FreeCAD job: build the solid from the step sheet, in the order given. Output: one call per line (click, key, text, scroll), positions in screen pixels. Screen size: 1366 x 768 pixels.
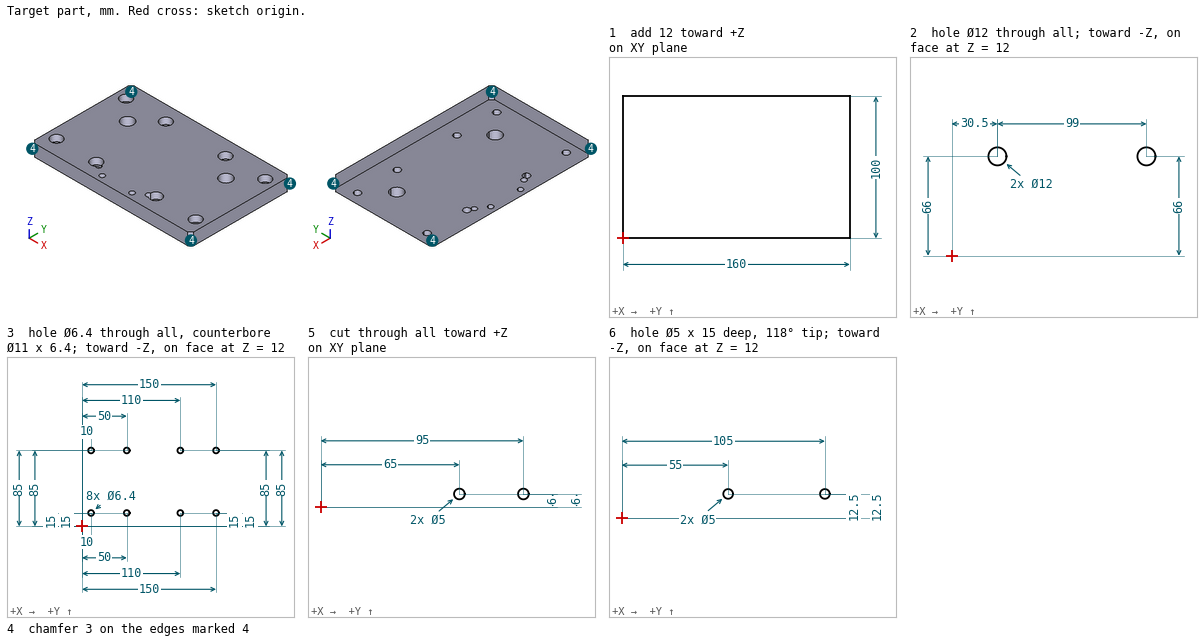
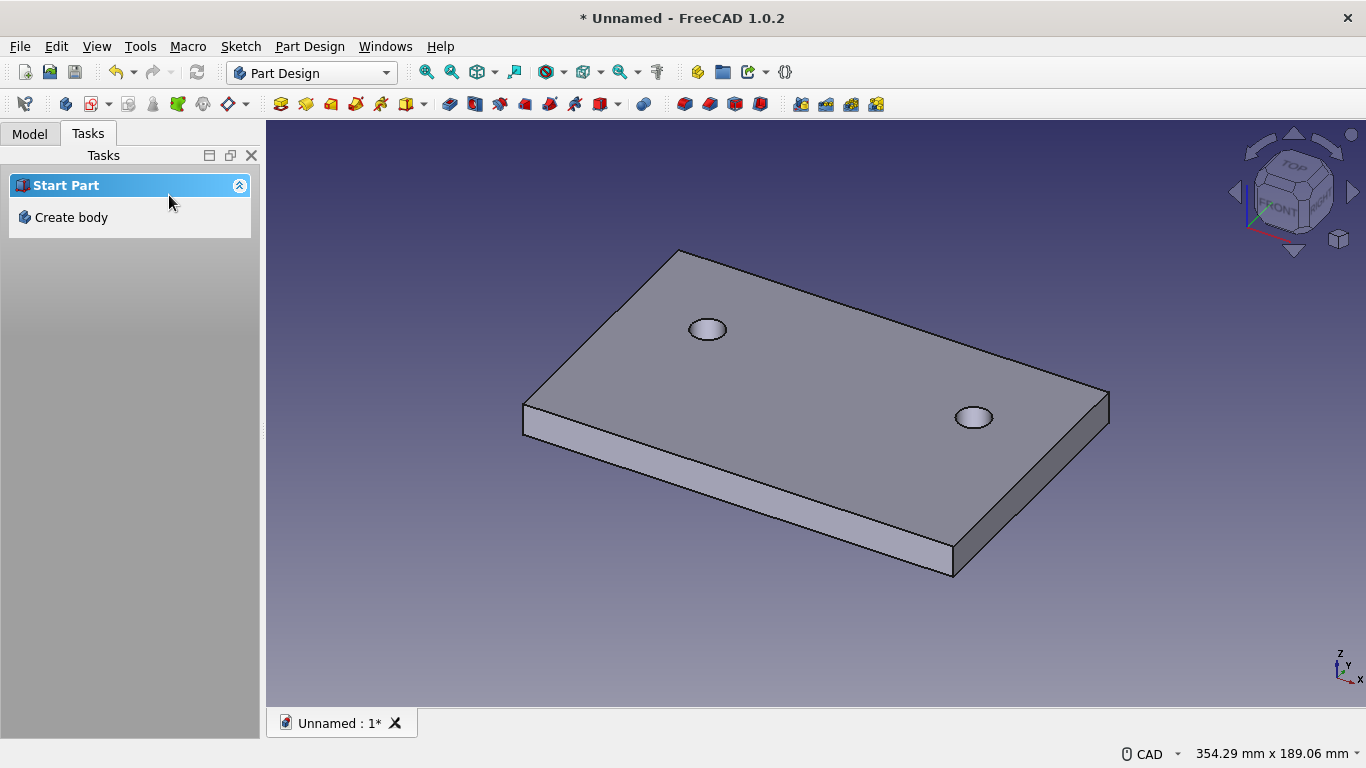
click(816, 397)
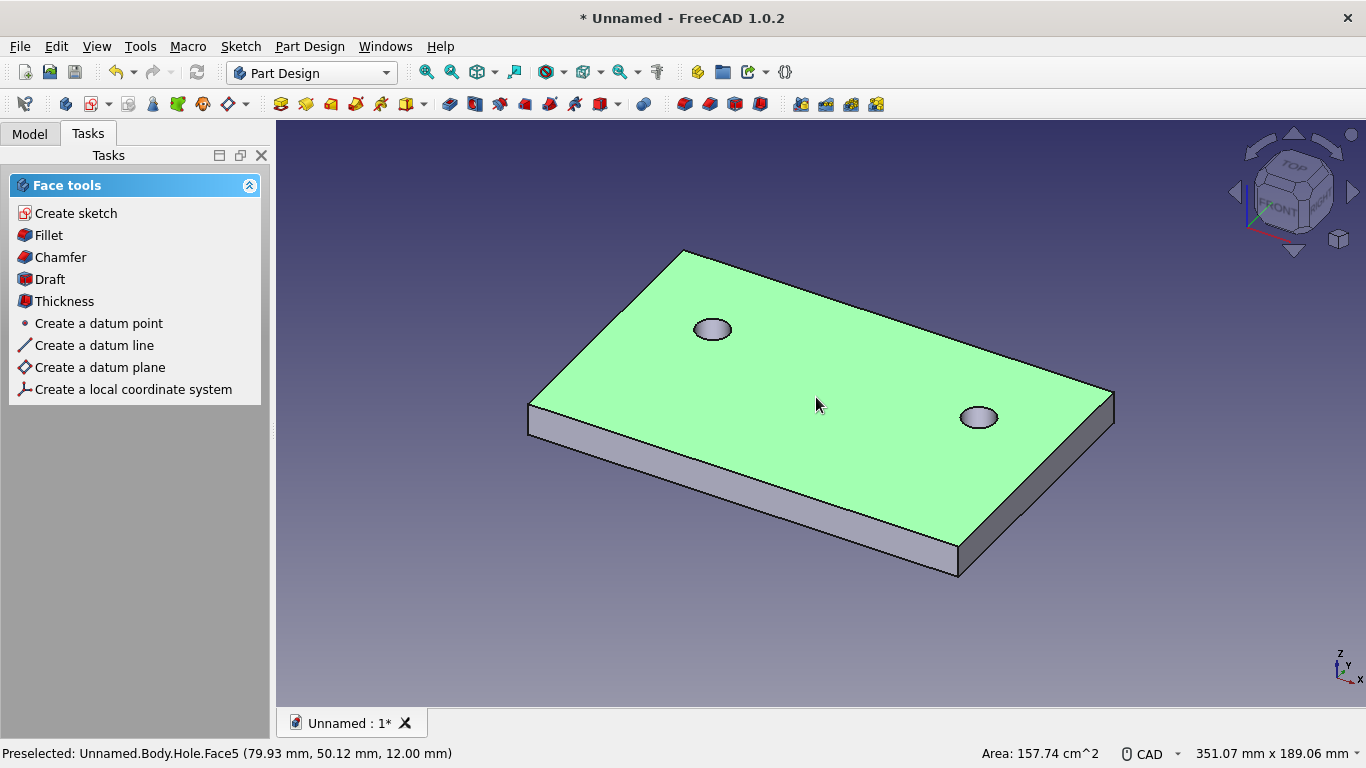
click(90, 104)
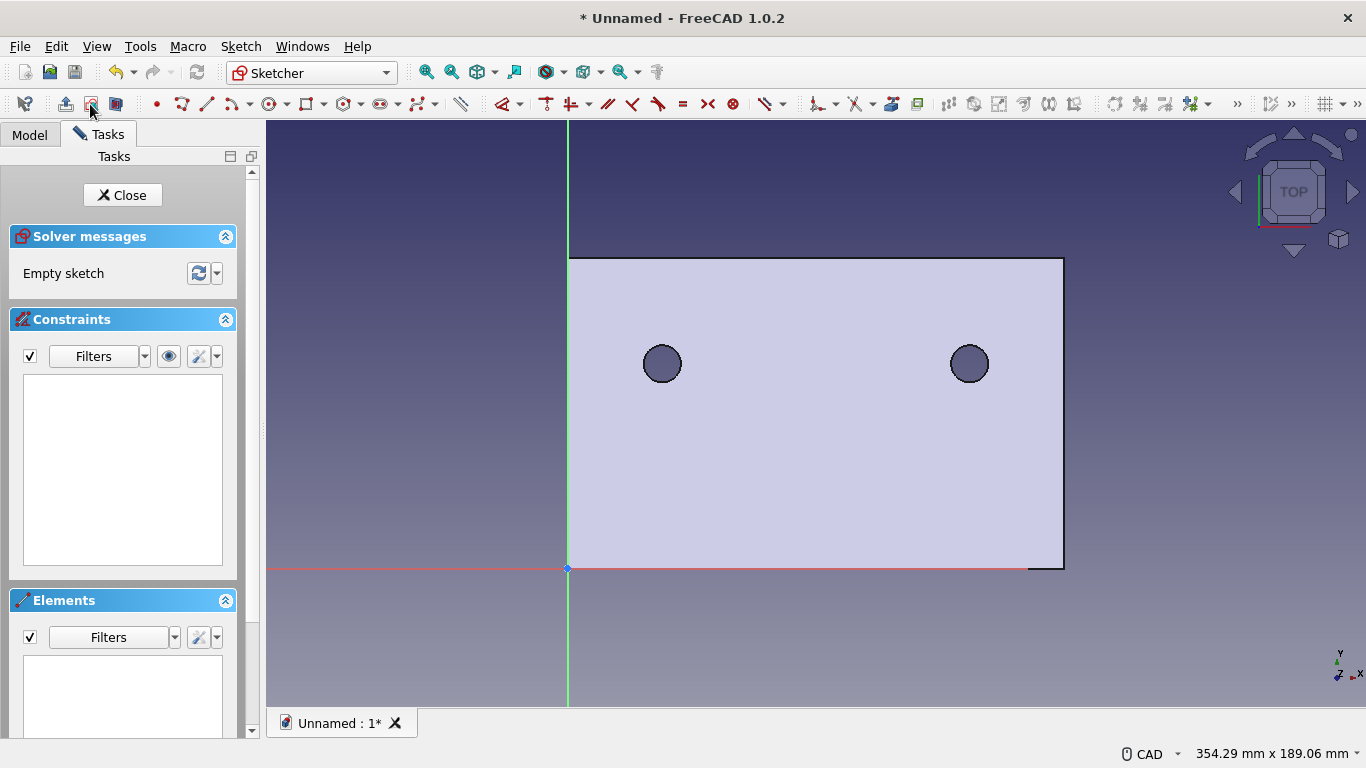
key(g)
key(c)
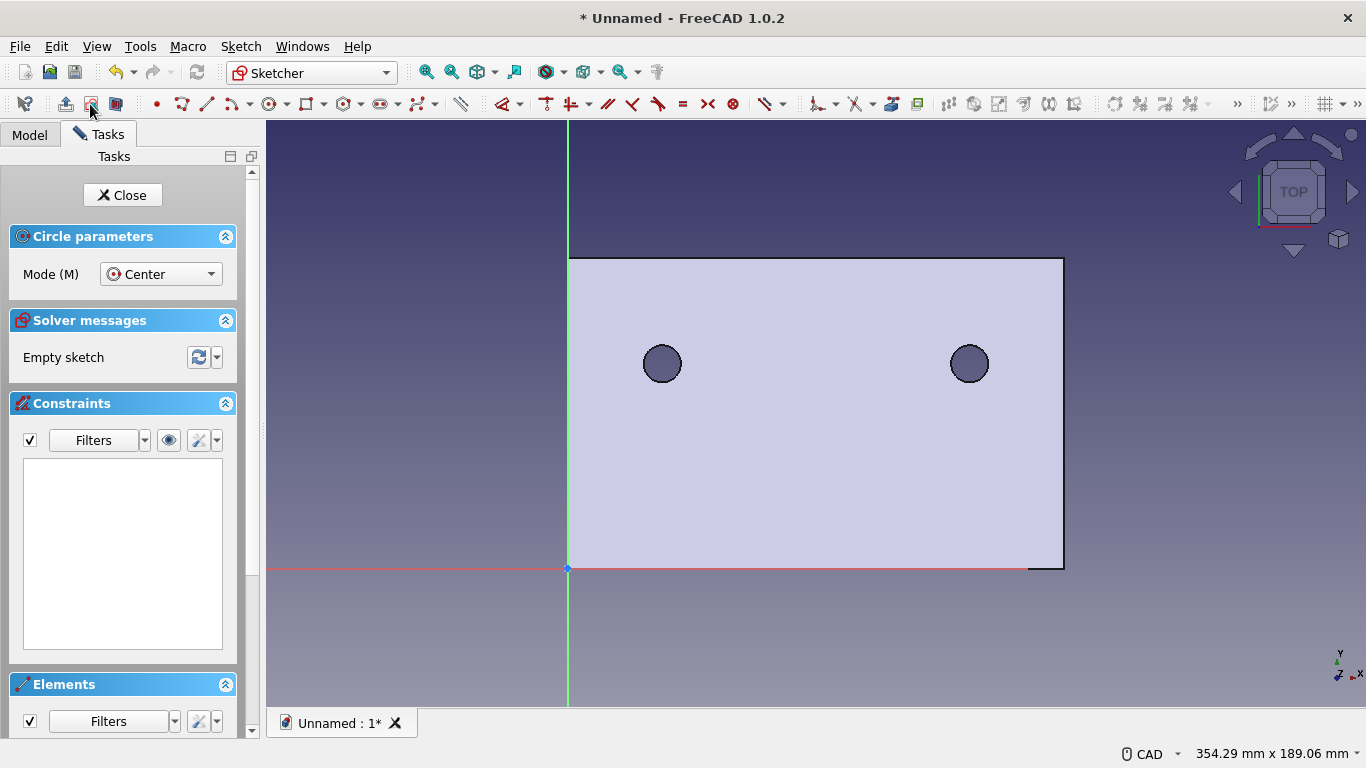
scroll(599, 522, up, 5)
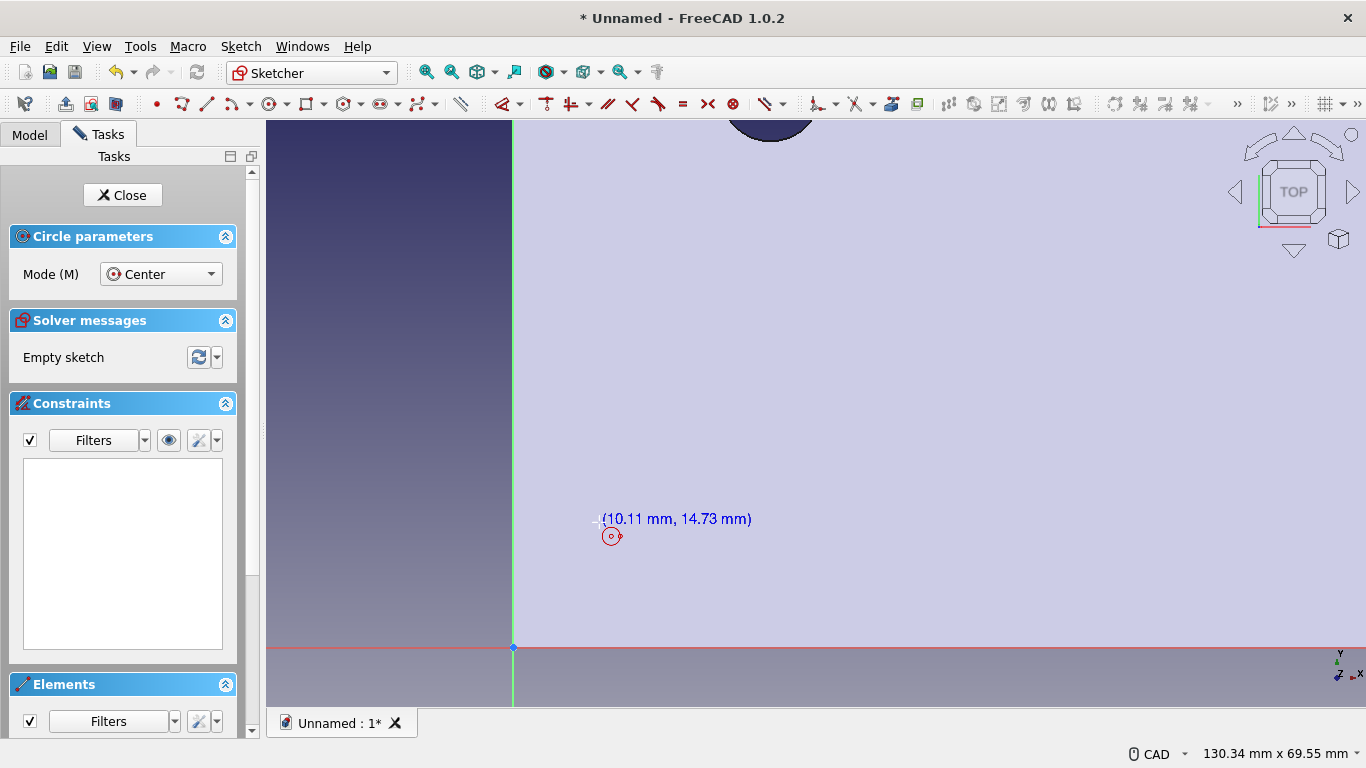
click(598, 521)
click(617, 502)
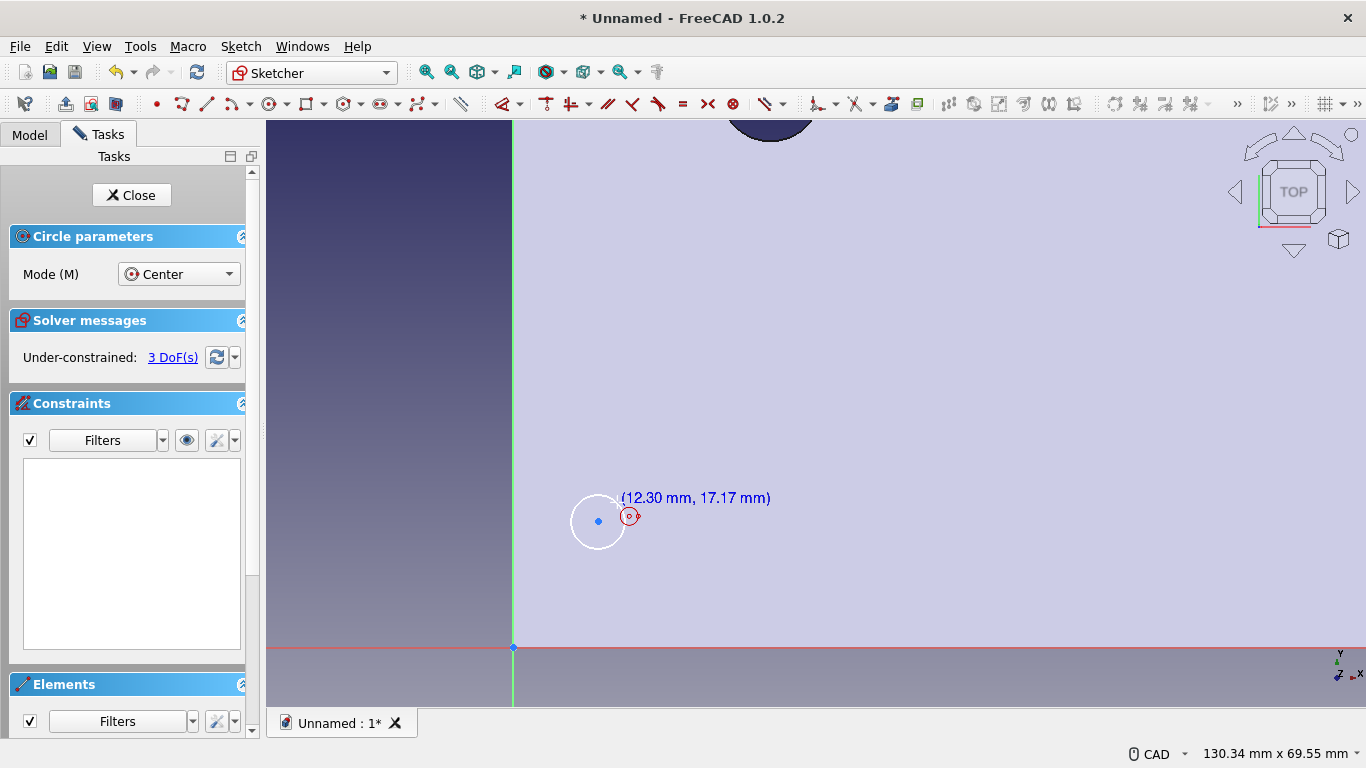
click(935, 521)
click(954, 502)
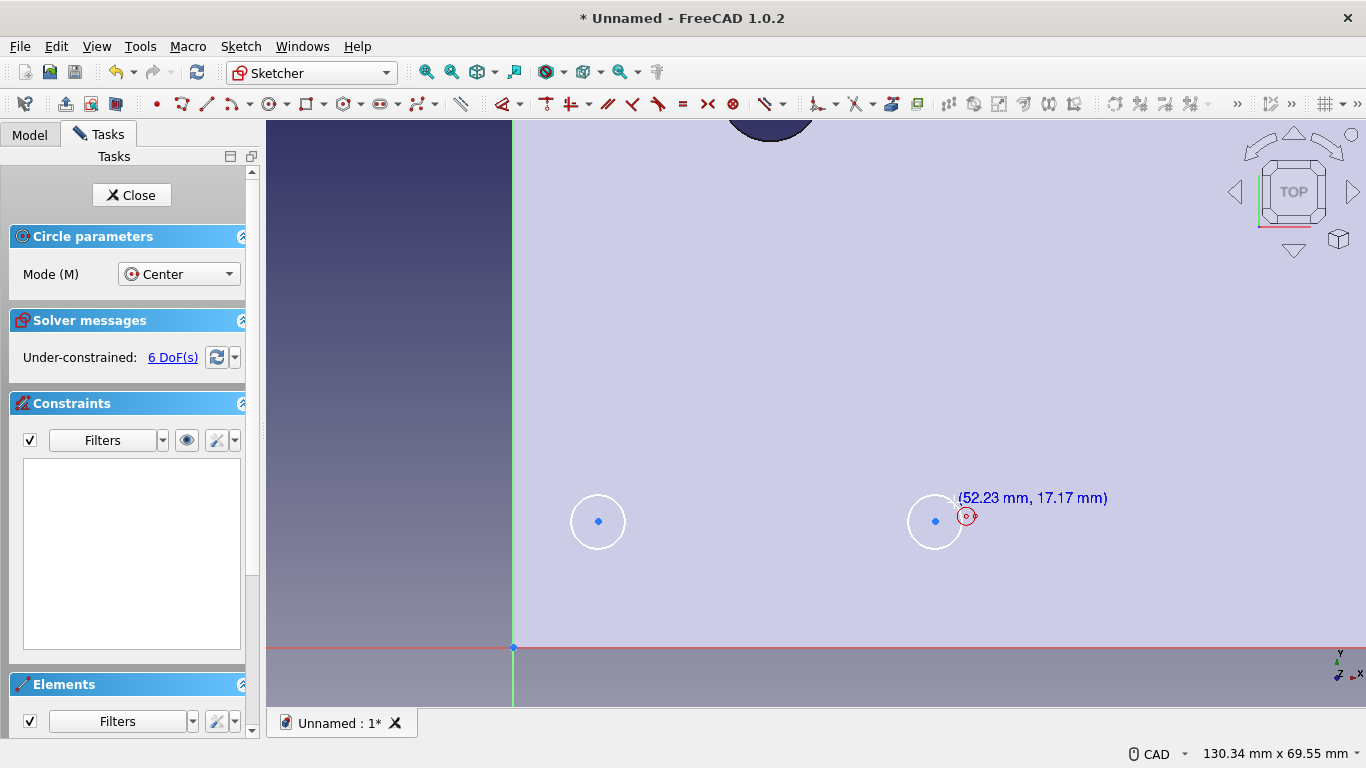
scroll(411, 526, down, 4)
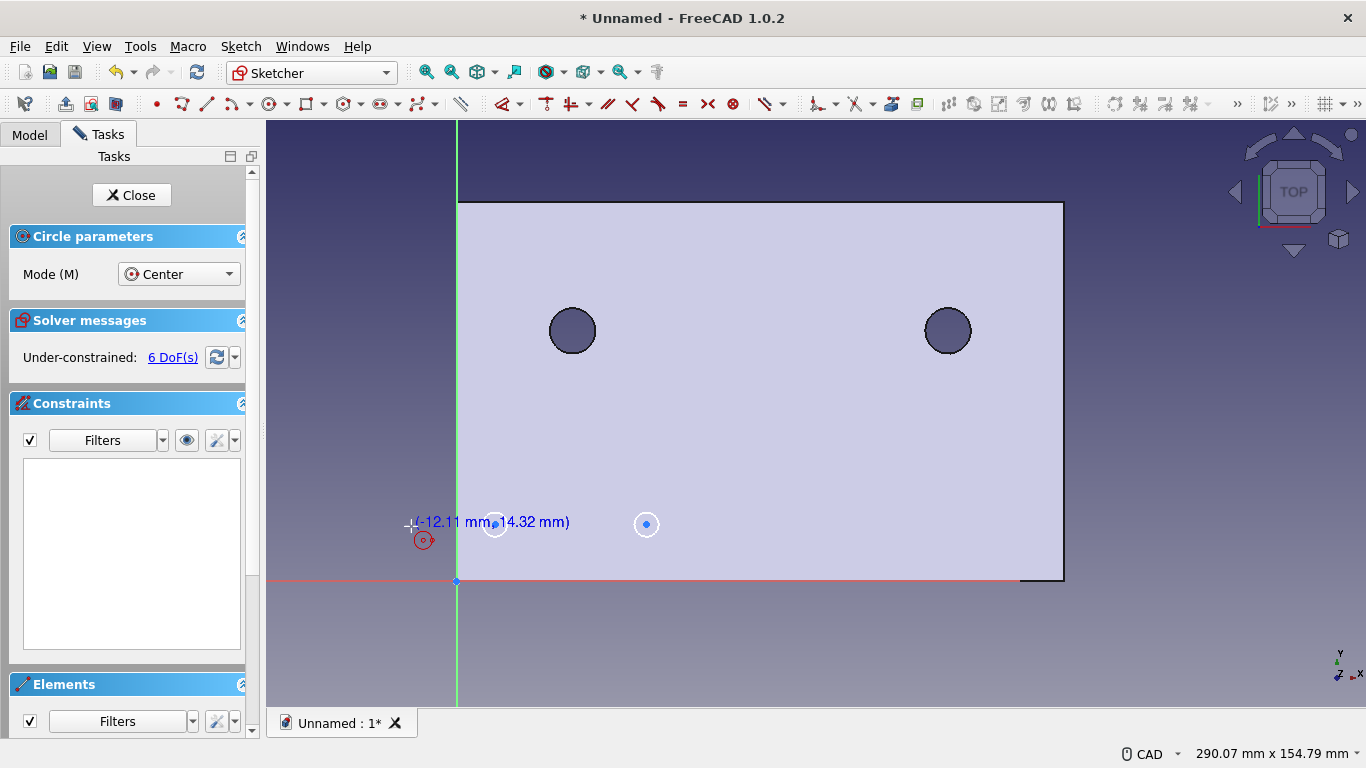
scroll(647, 259, up, 4)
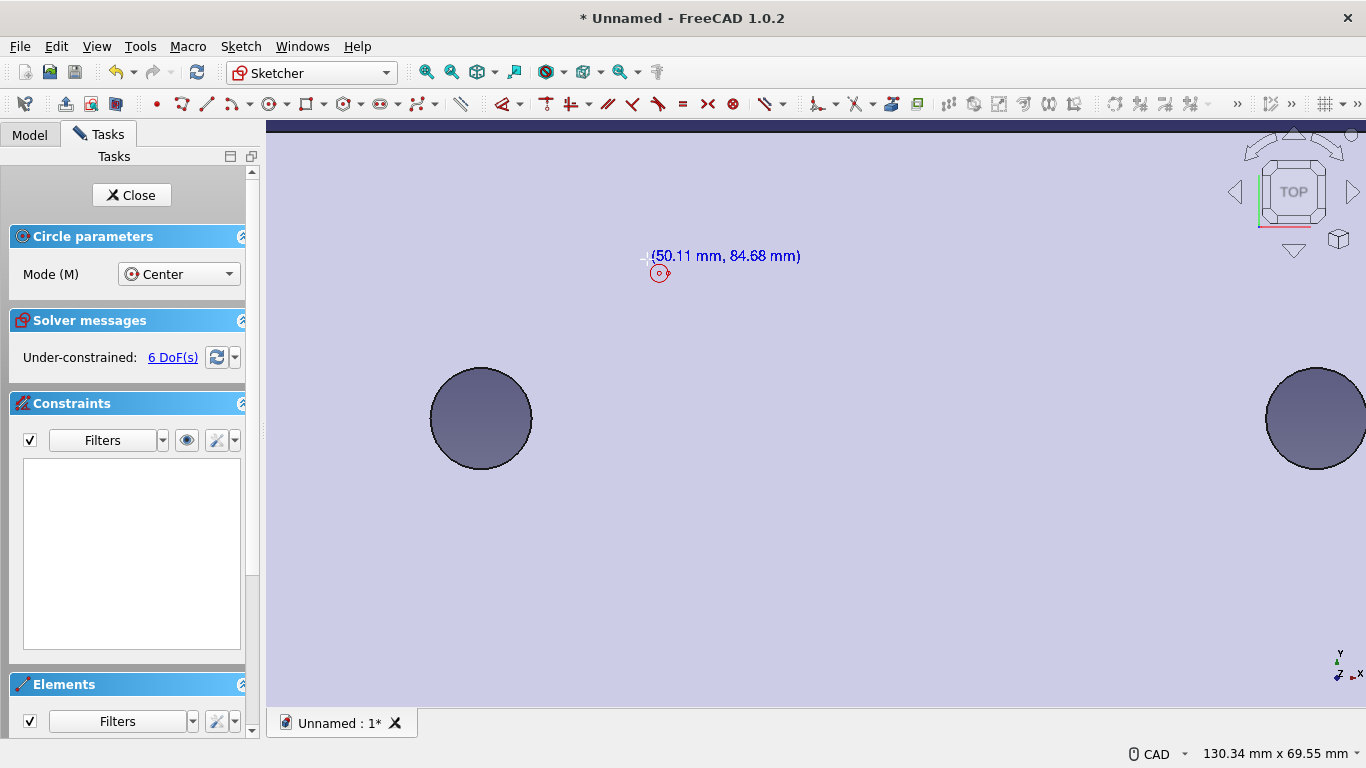
click(646, 258)
click(665, 239)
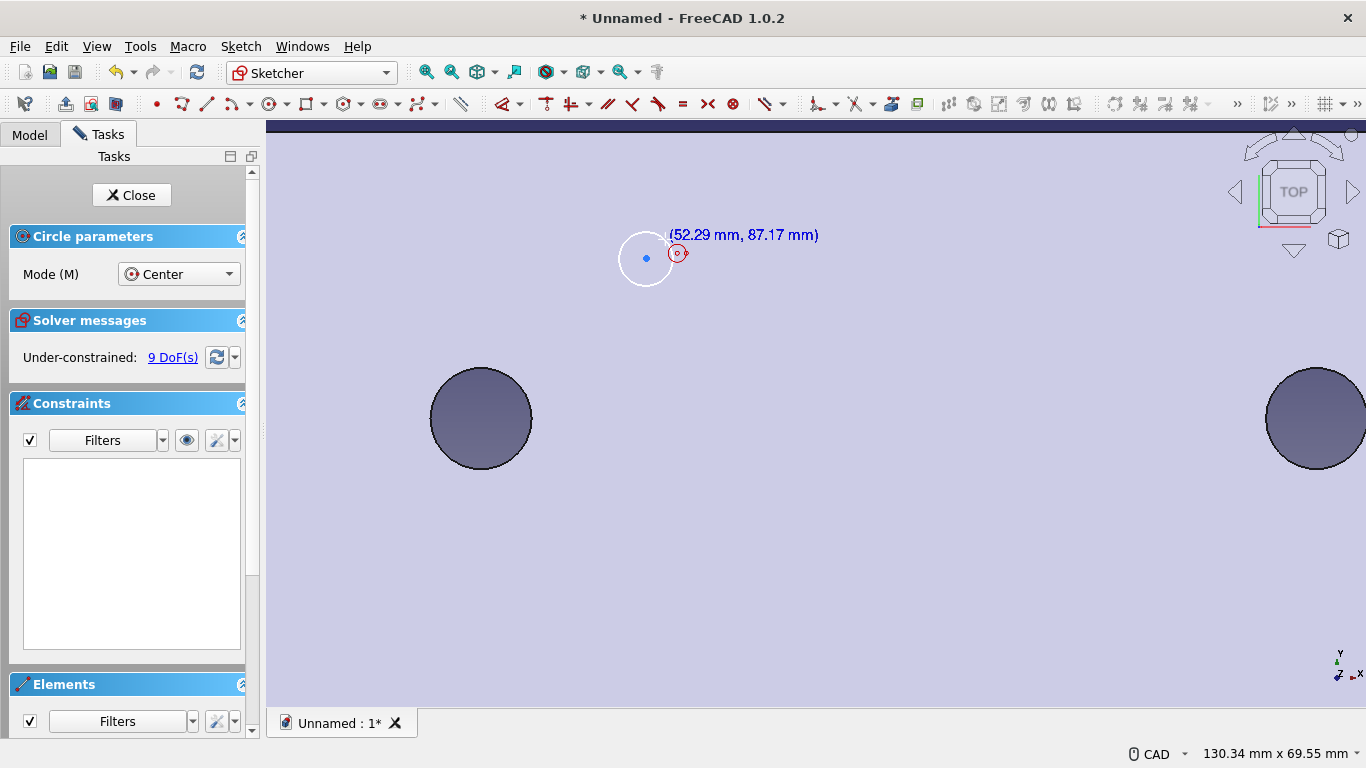
click(308, 258)
click(327, 239)